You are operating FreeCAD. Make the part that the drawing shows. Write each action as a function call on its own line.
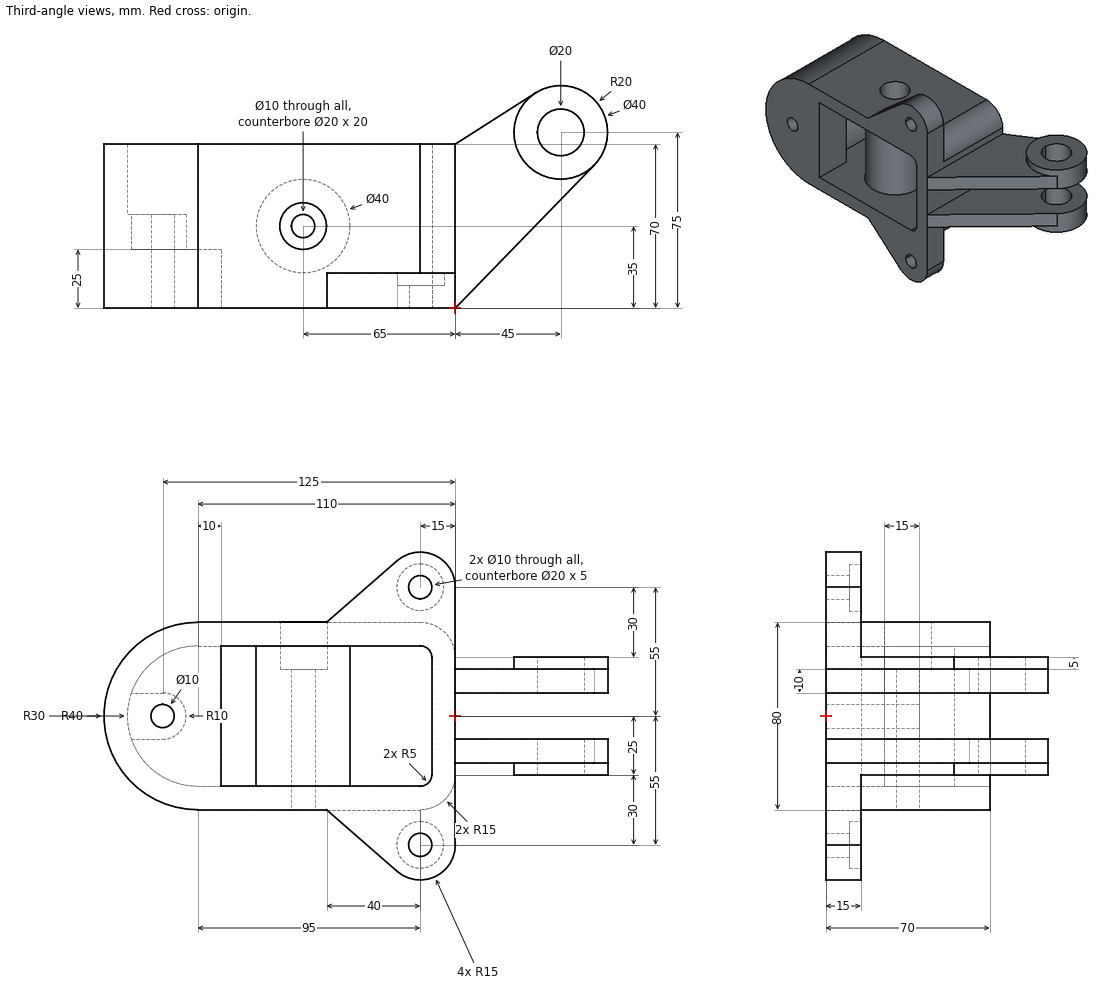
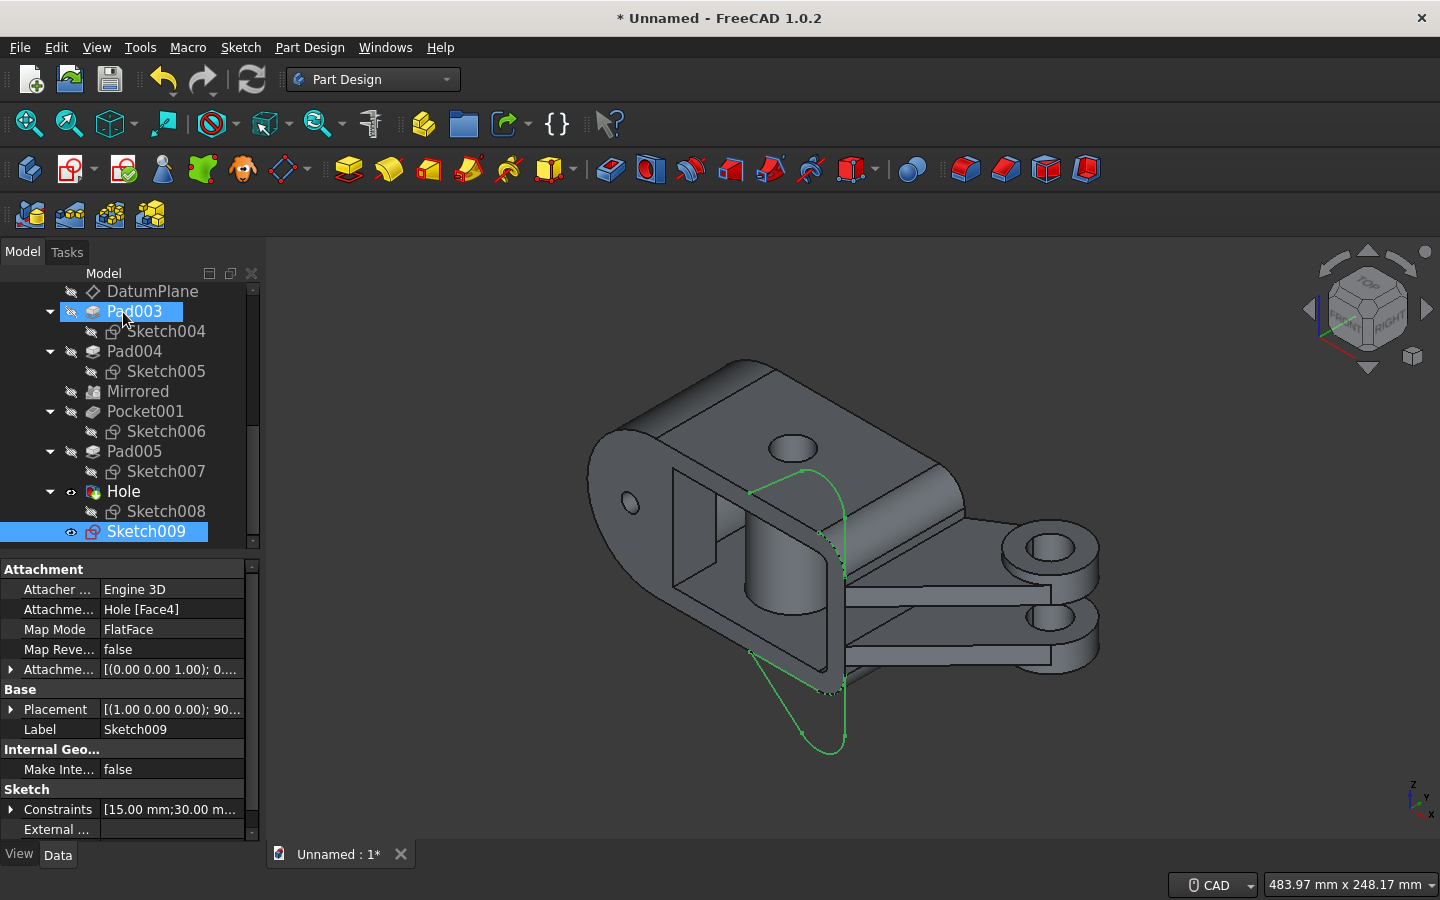
click(350, 170)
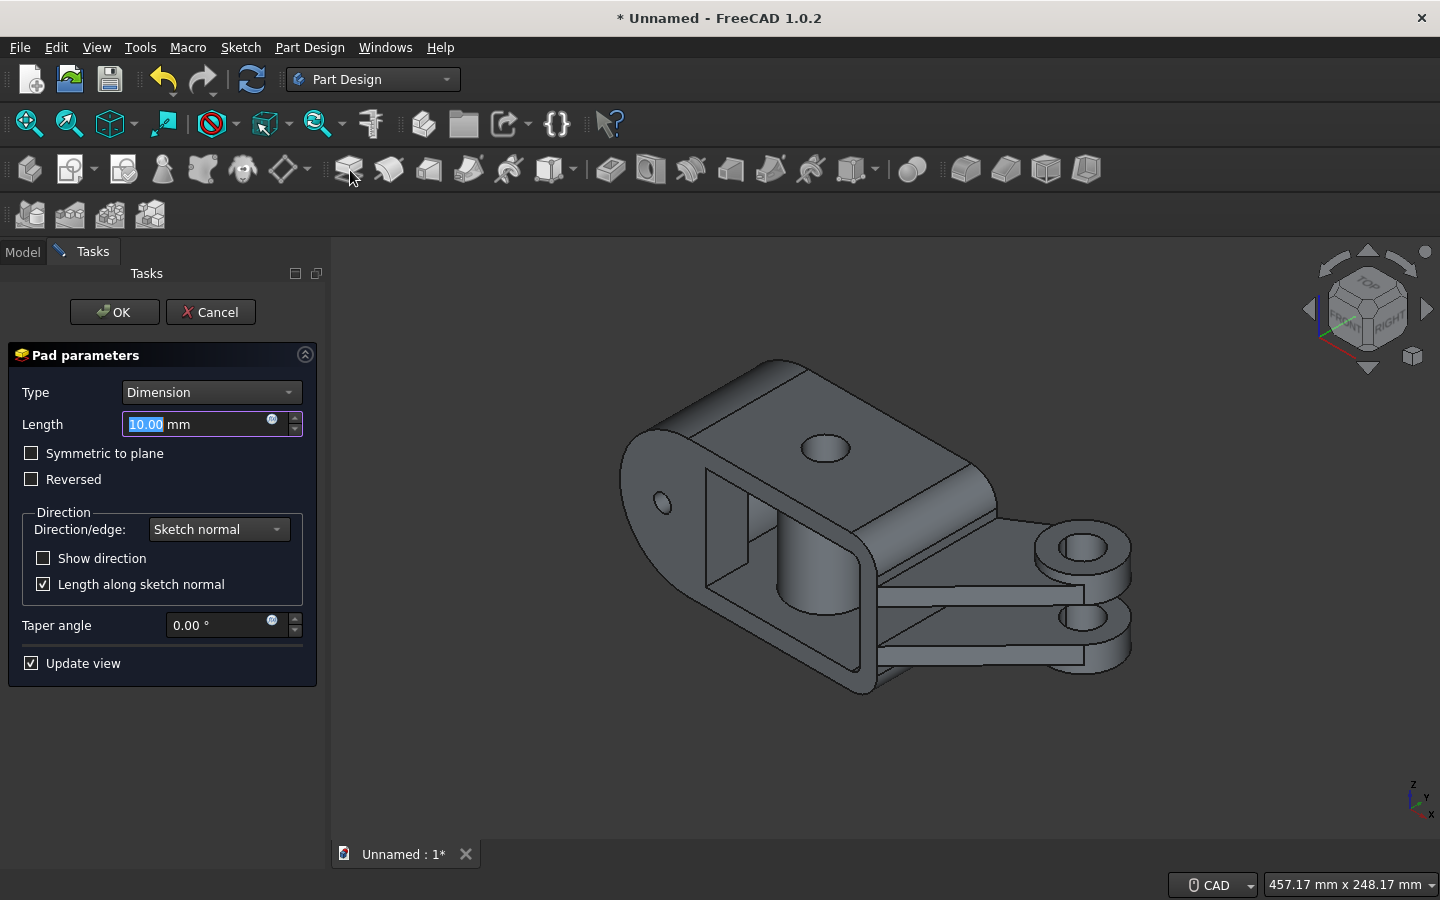
text(15)
key(Tab)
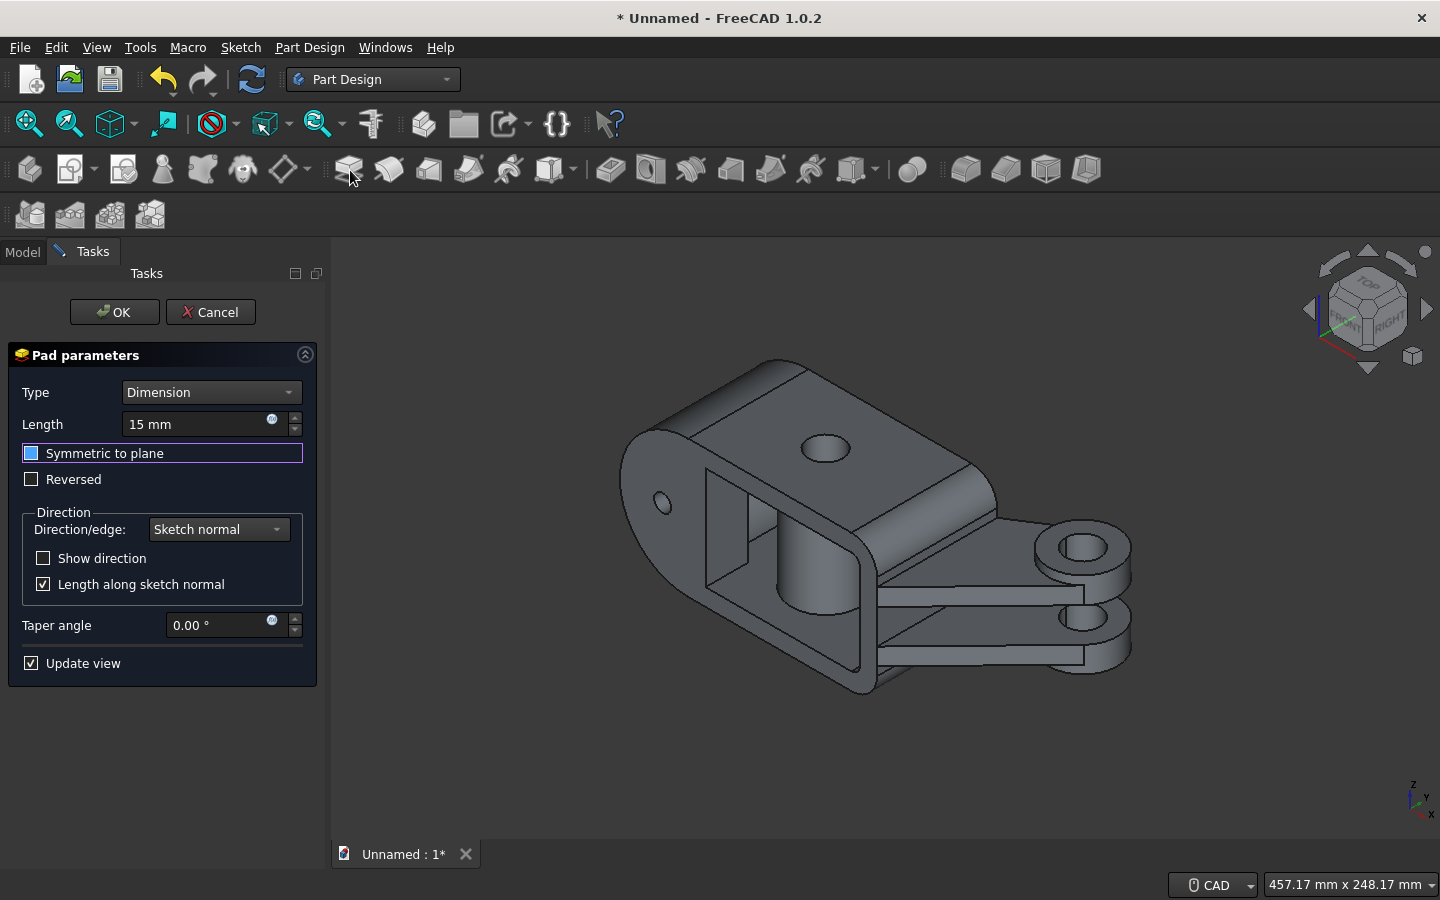
click(30, 479)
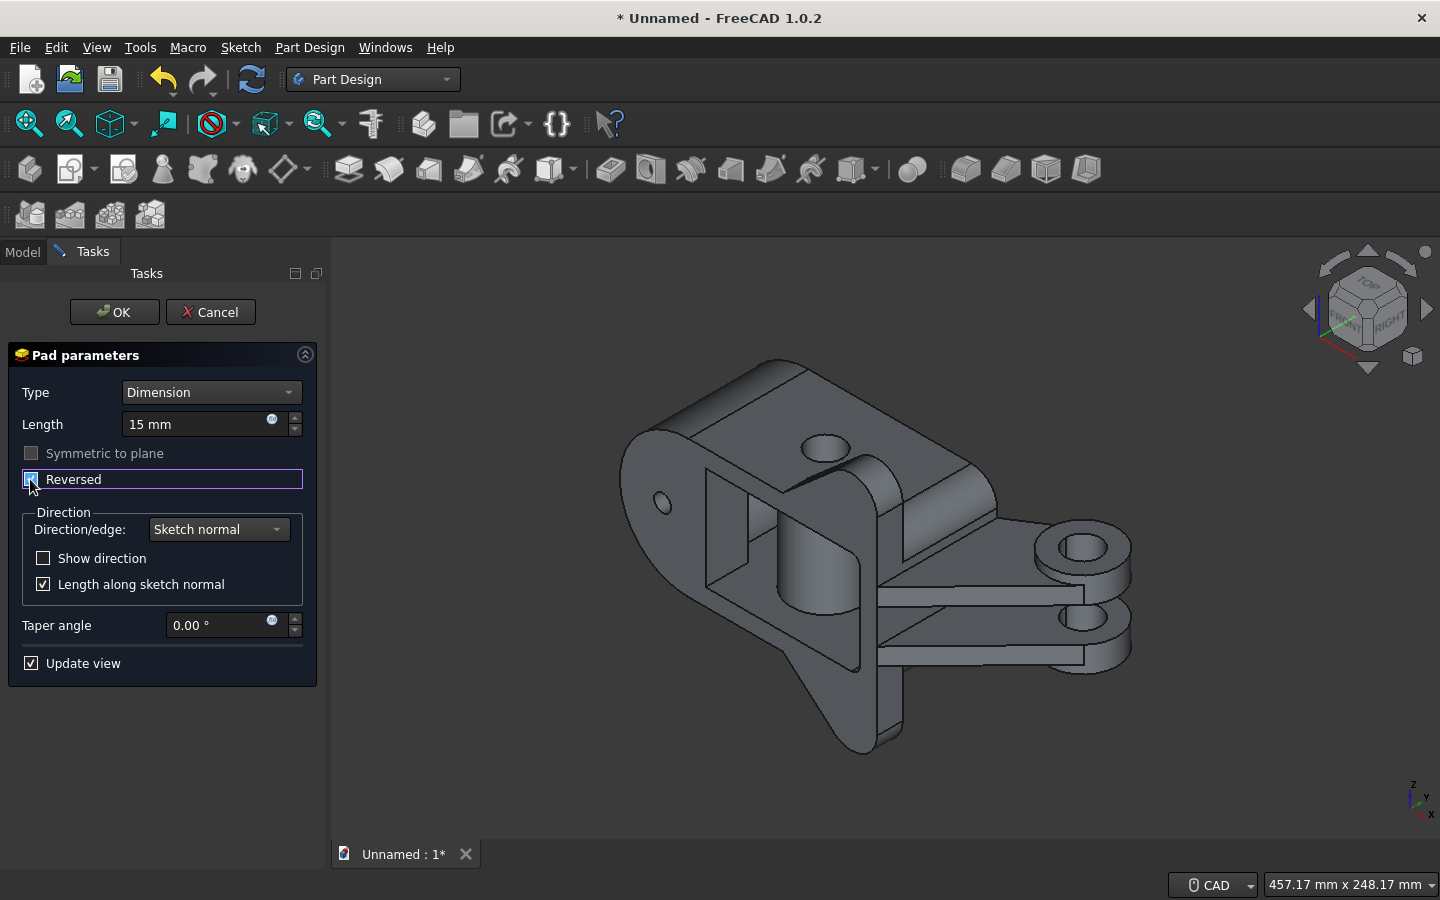
click(115, 312)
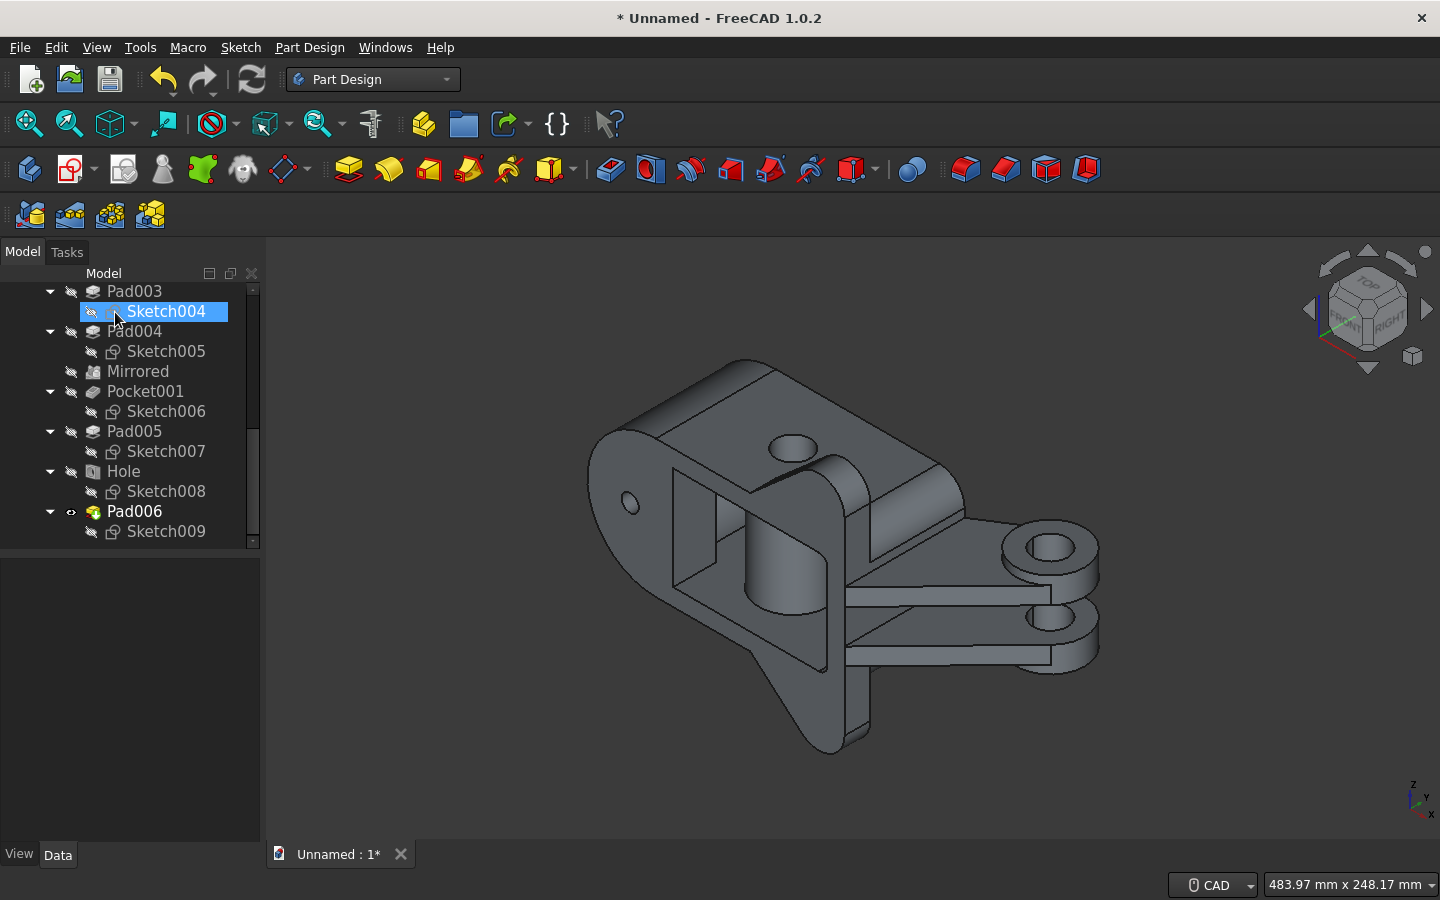
key(4)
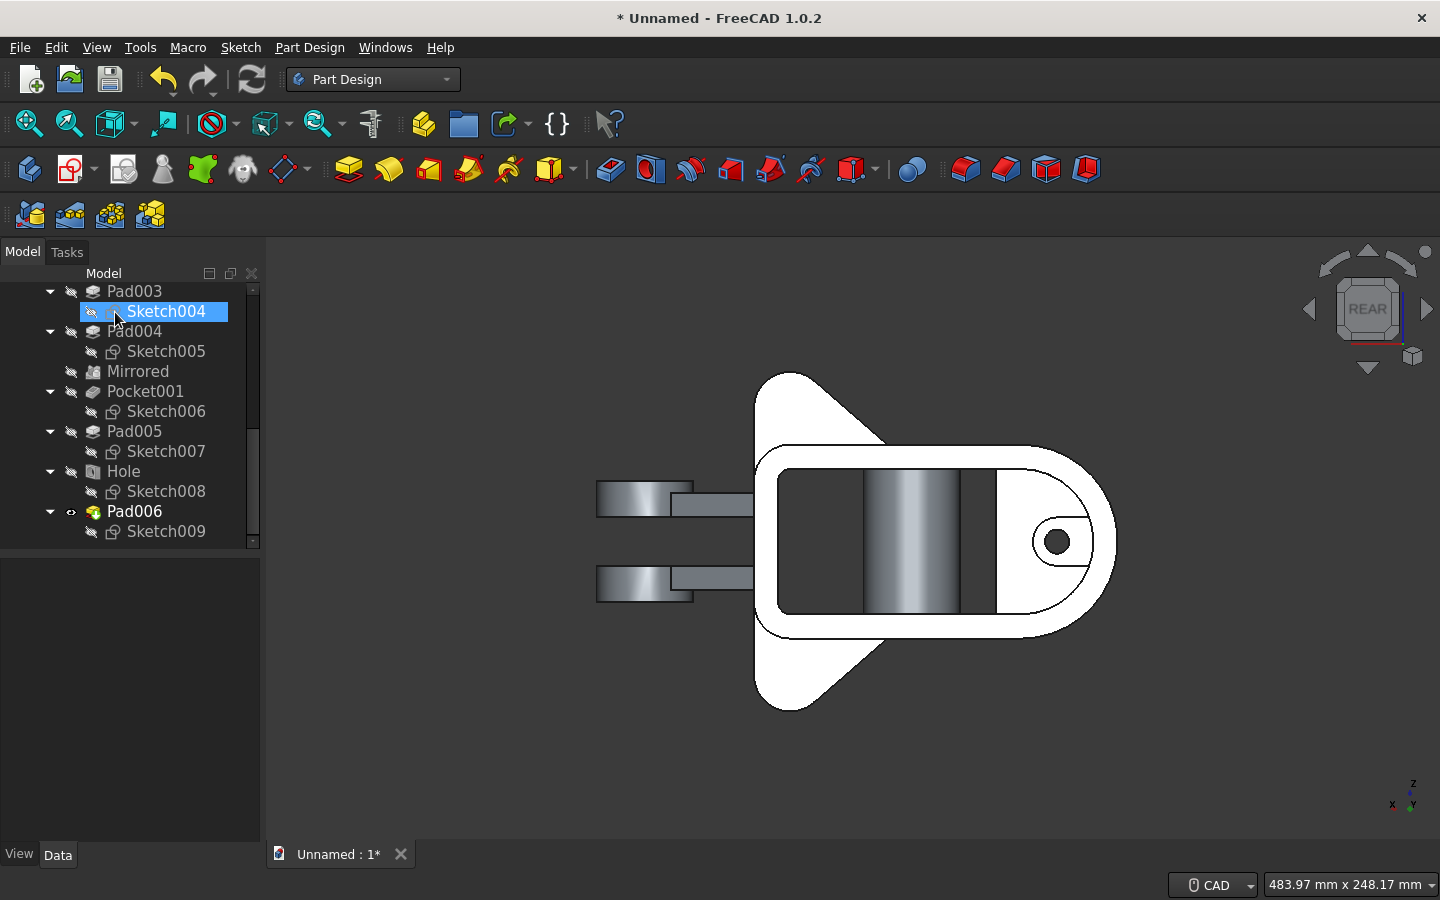
click(802, 410)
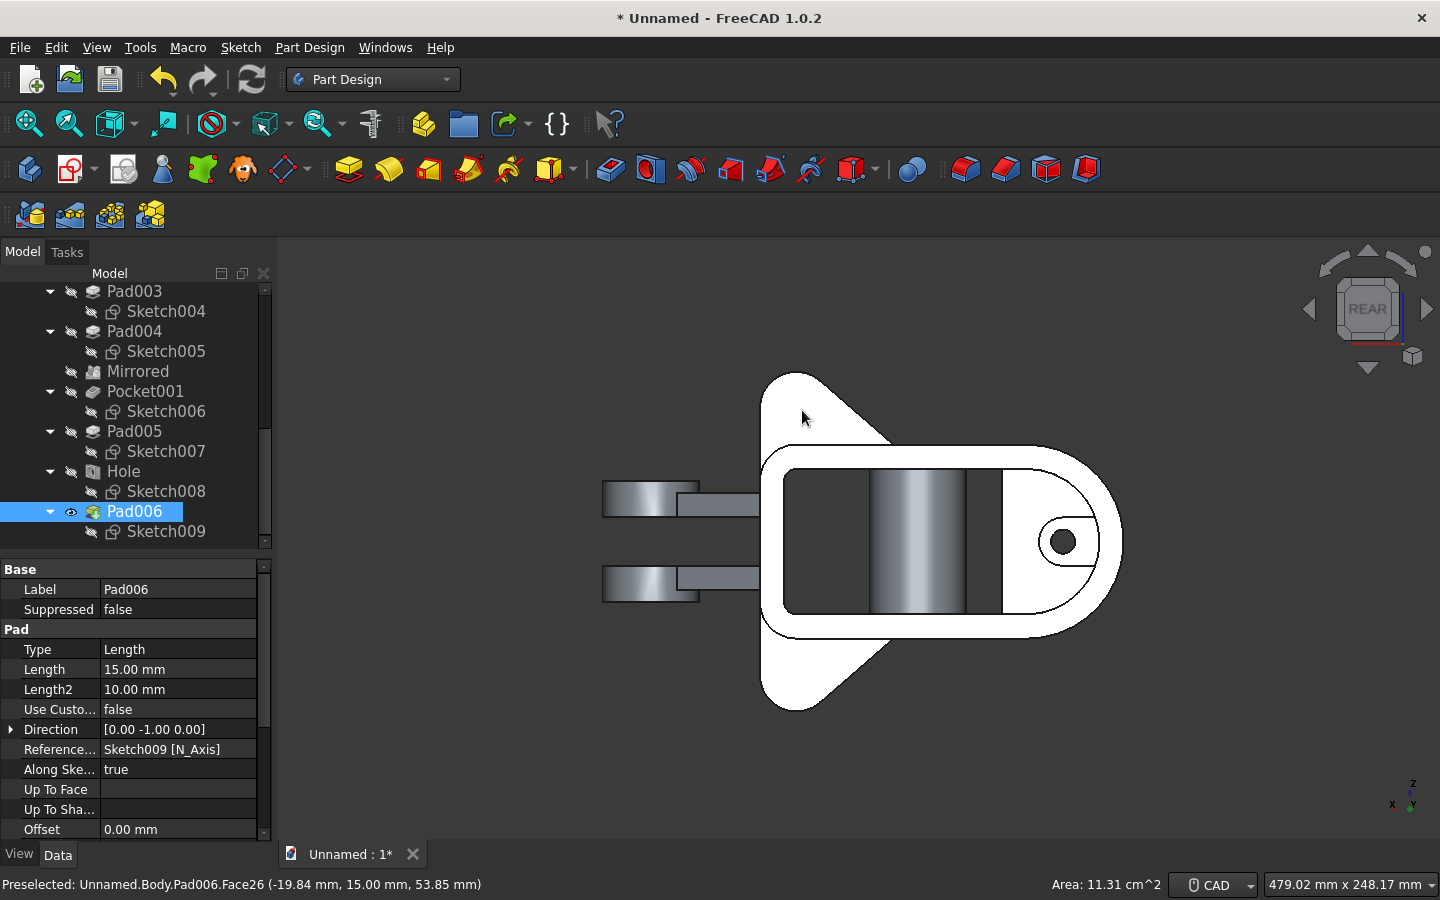
click(70, 170)